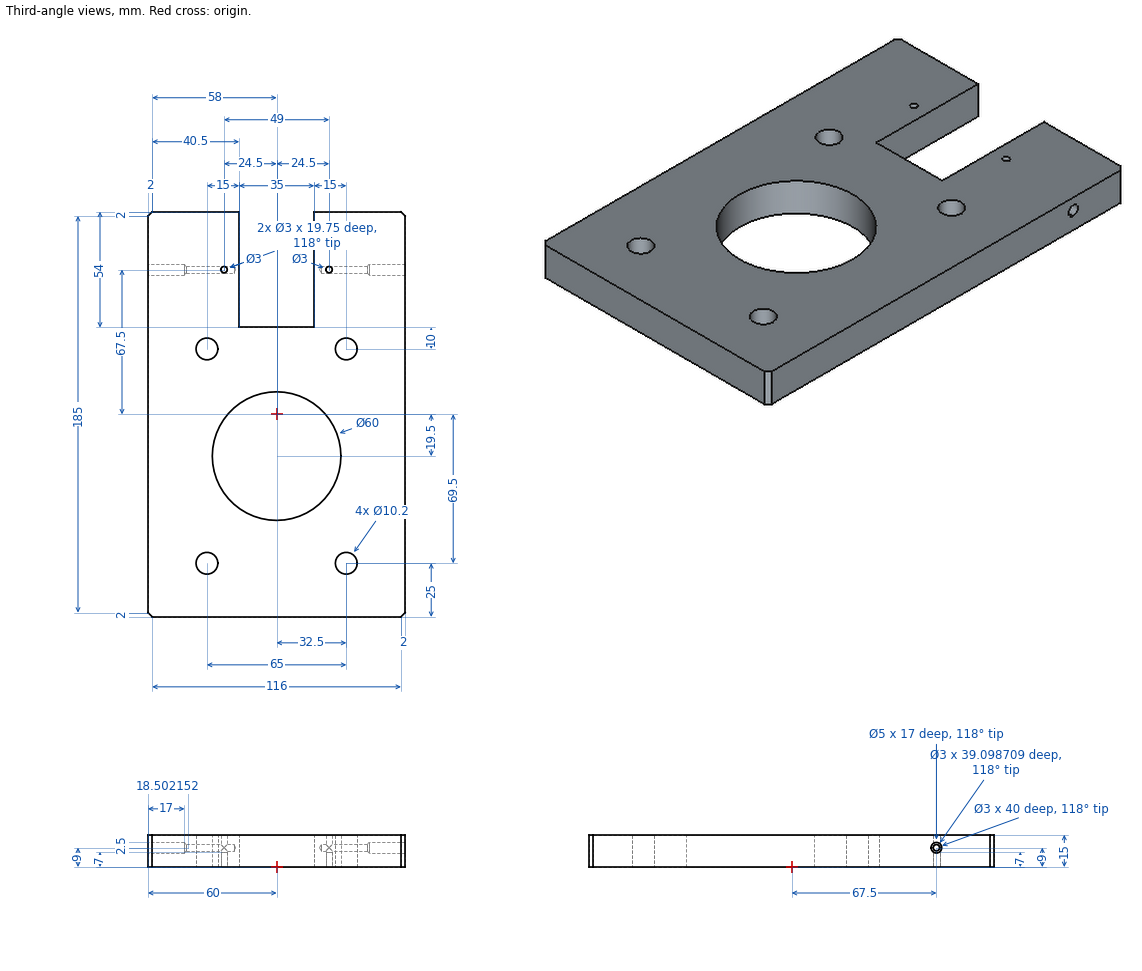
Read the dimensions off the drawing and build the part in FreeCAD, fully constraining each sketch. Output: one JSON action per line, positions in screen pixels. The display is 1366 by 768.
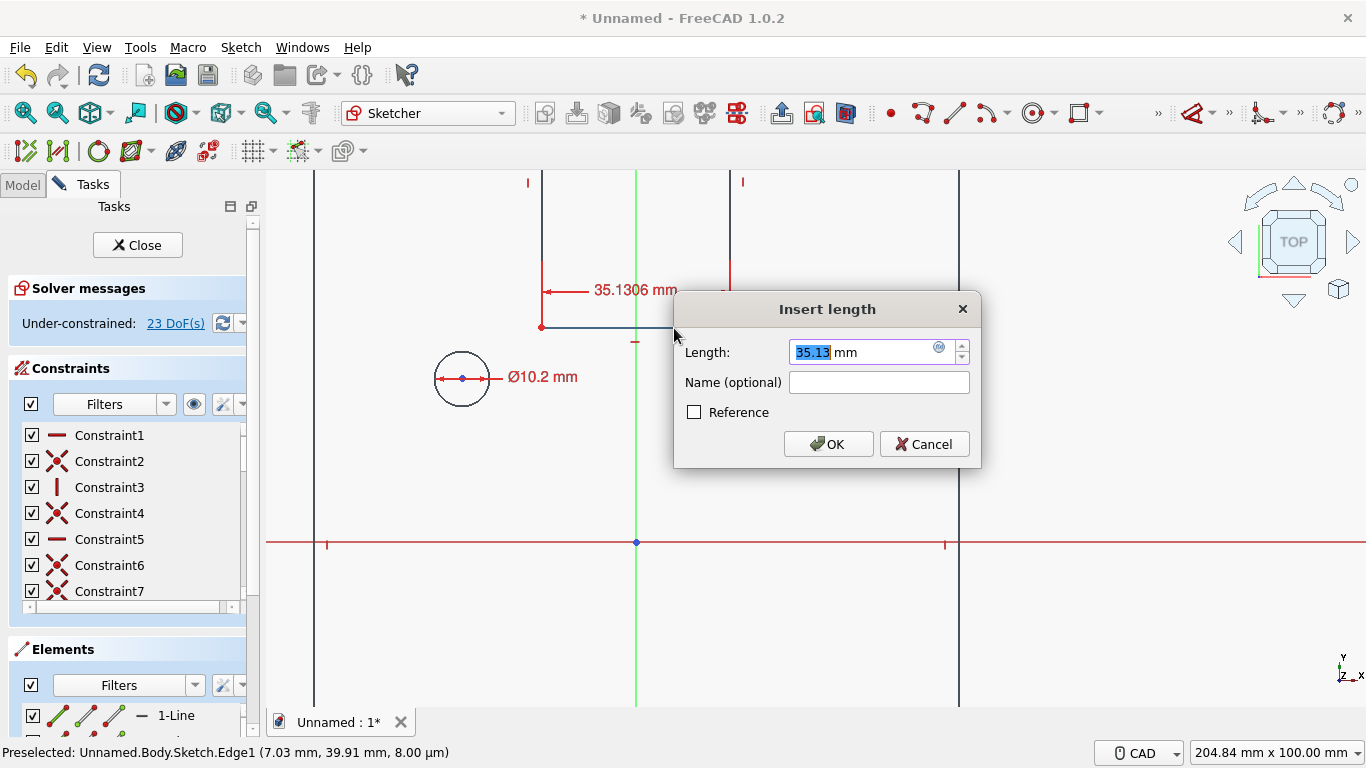
{"action": "type", "text": "35"}
{"action": "key", "text": "Return"}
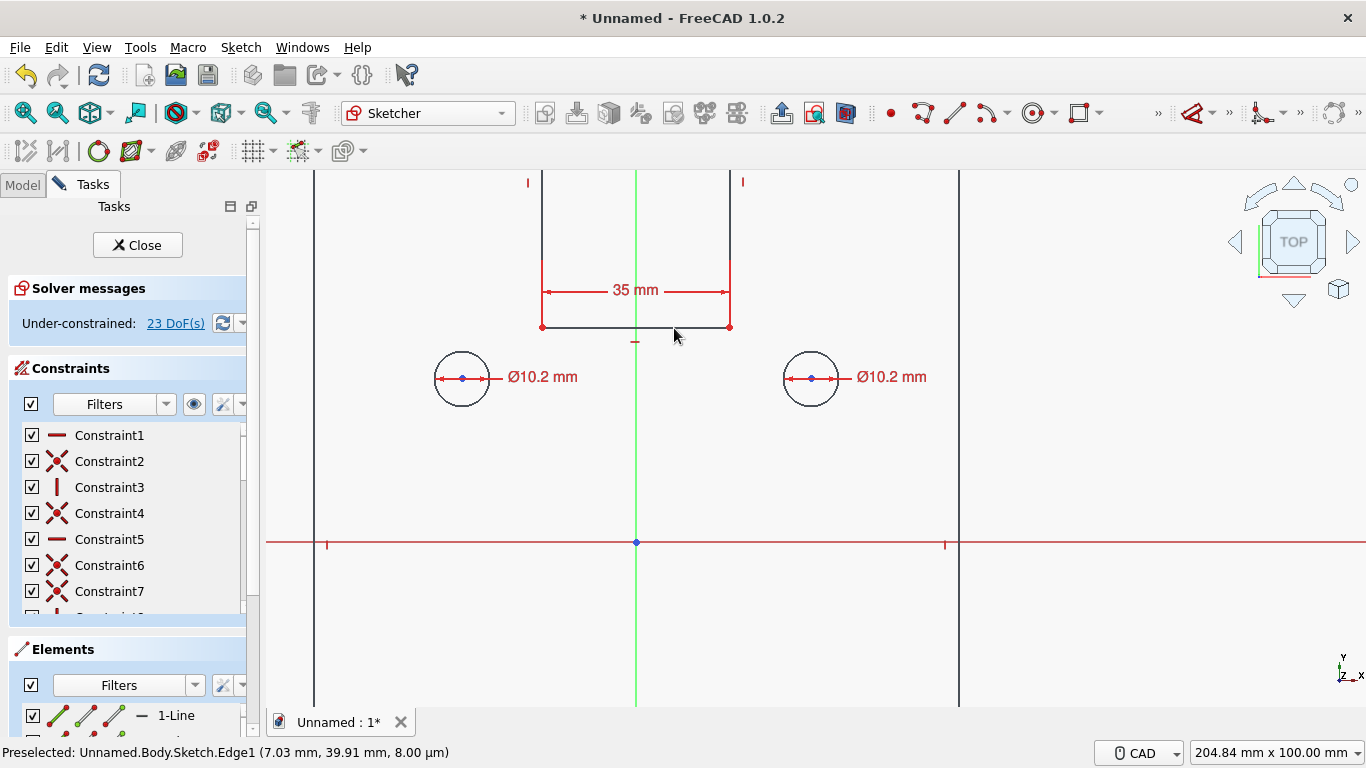
{"action": "left_click", "coordinate": [542, 241]}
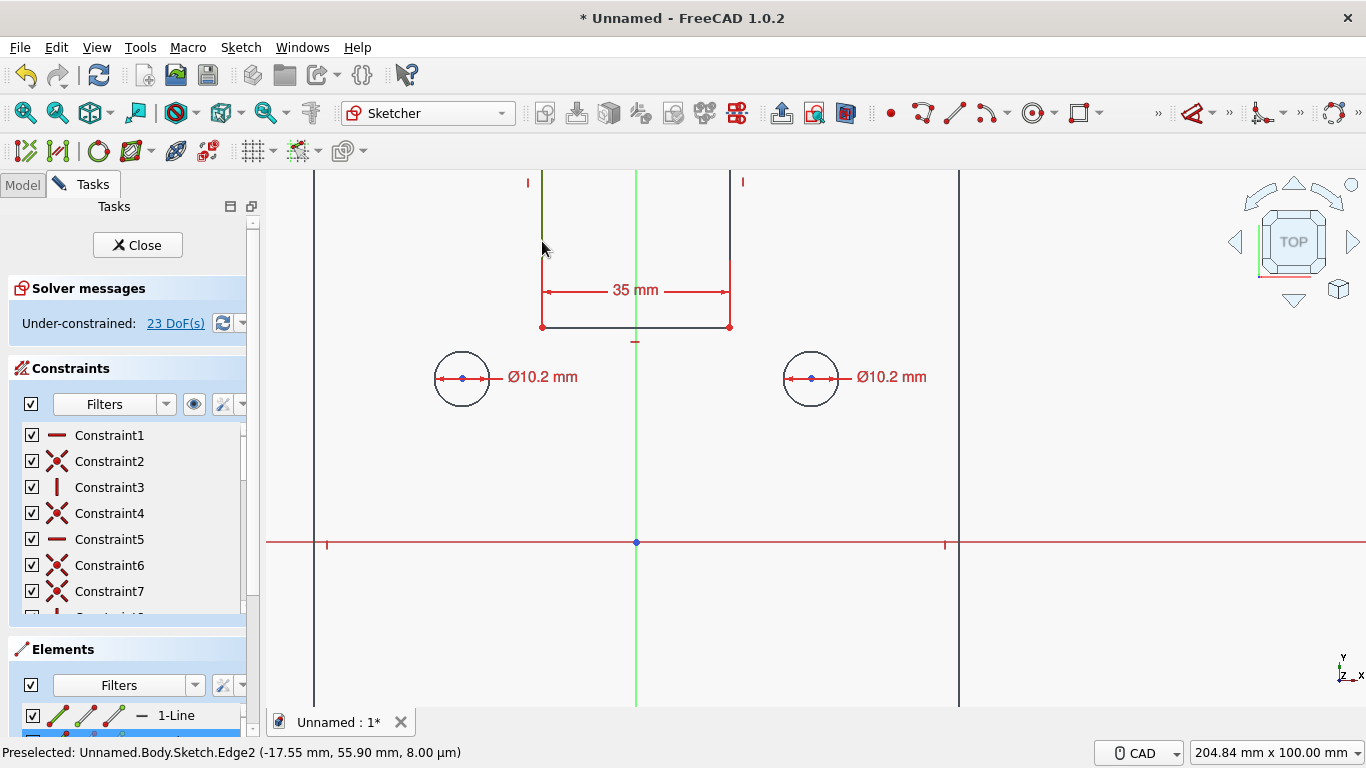
{"action": "key", "text": "i"}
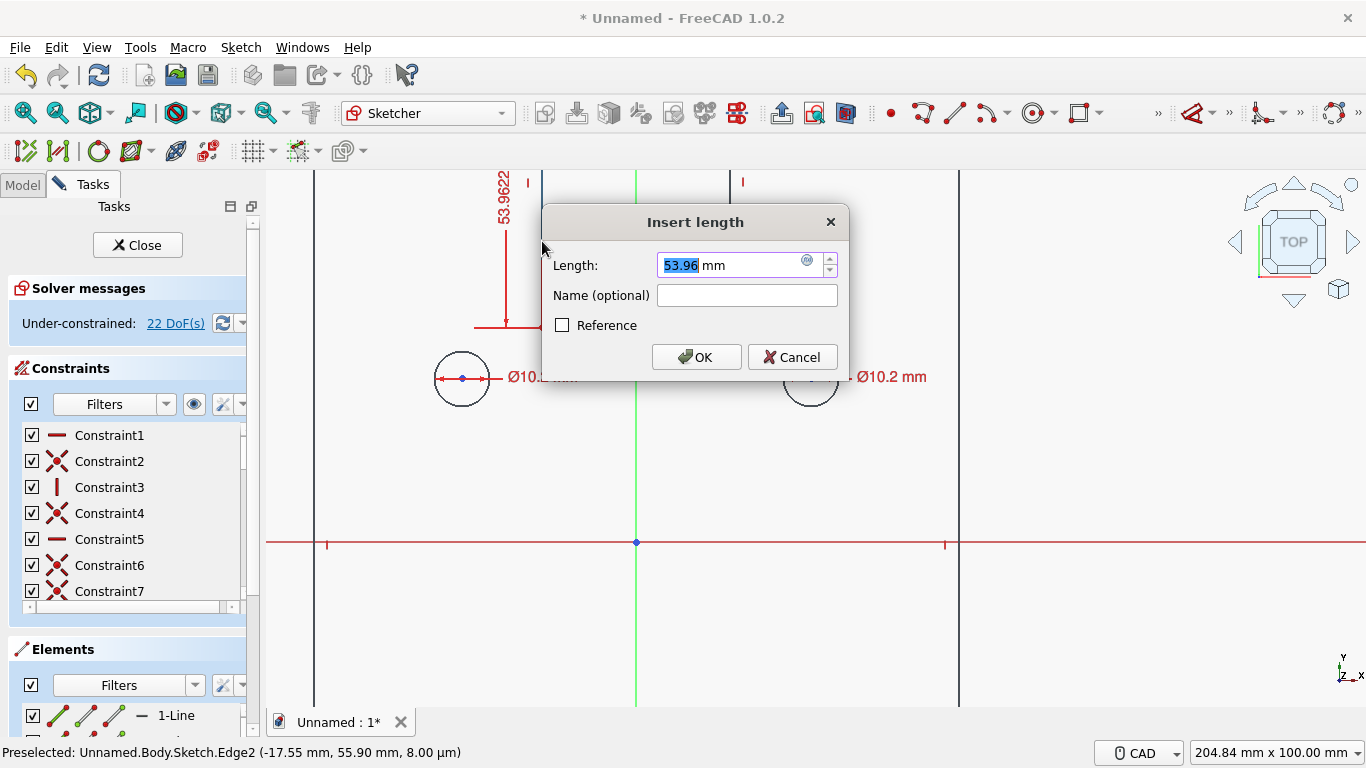
{"action": "type", "text": "54"}
{"action": "key", "text": "Return"}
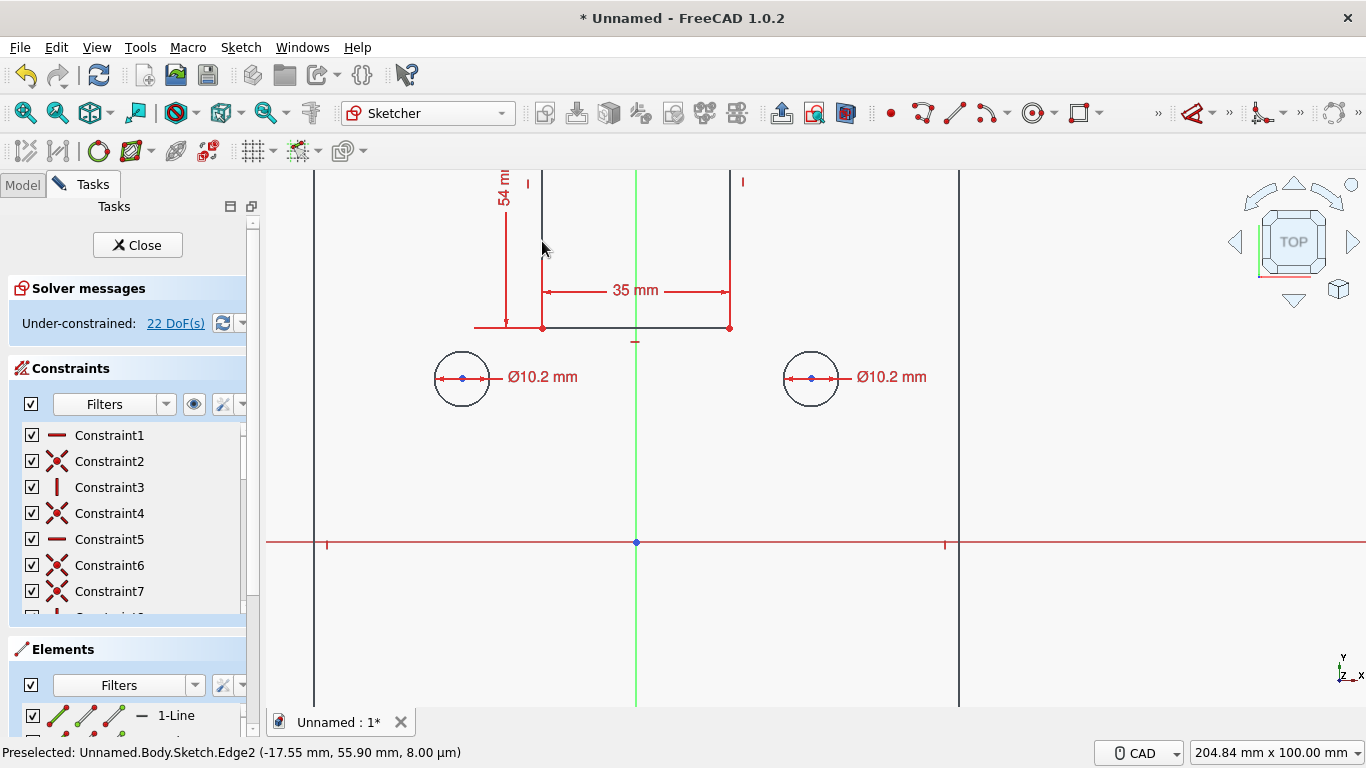
{"action": "left_click", "coordinate": [730, 240]}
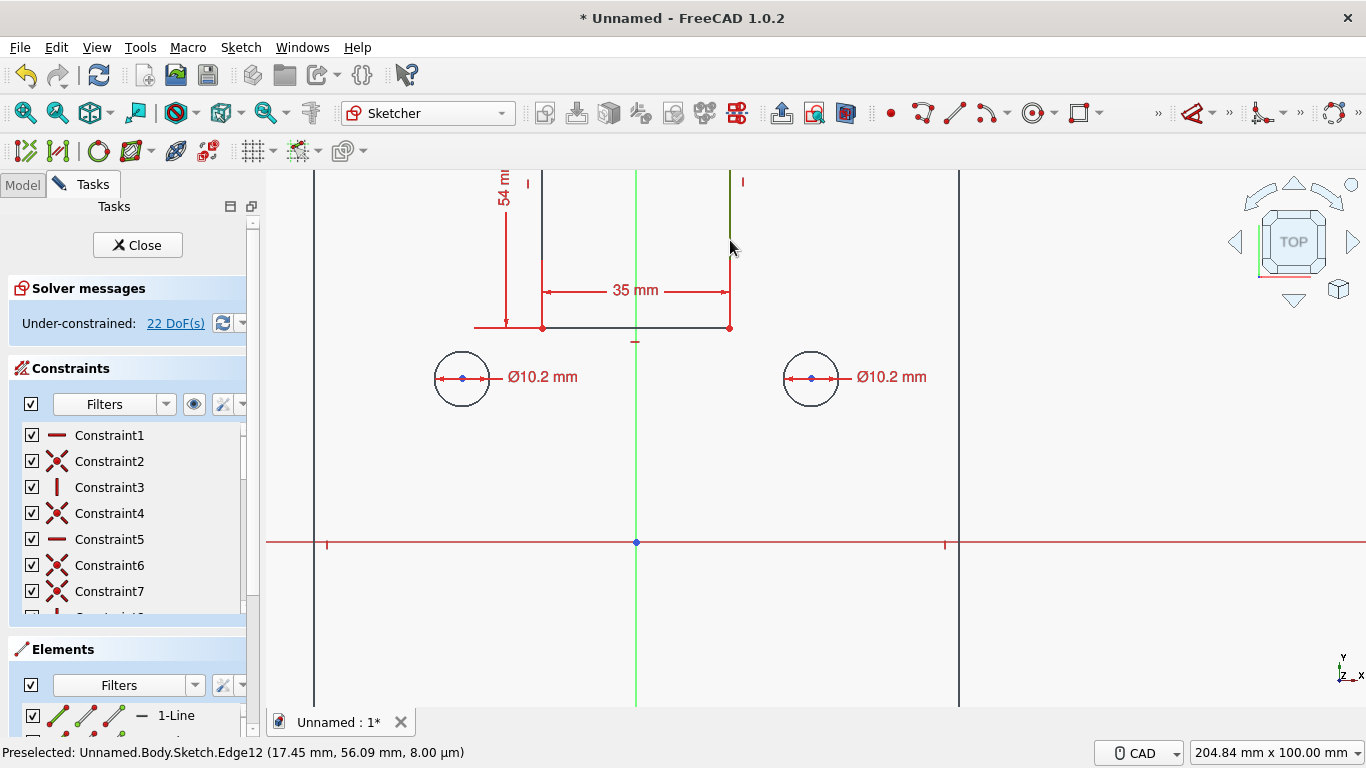
{"action": "key", "text": "i"}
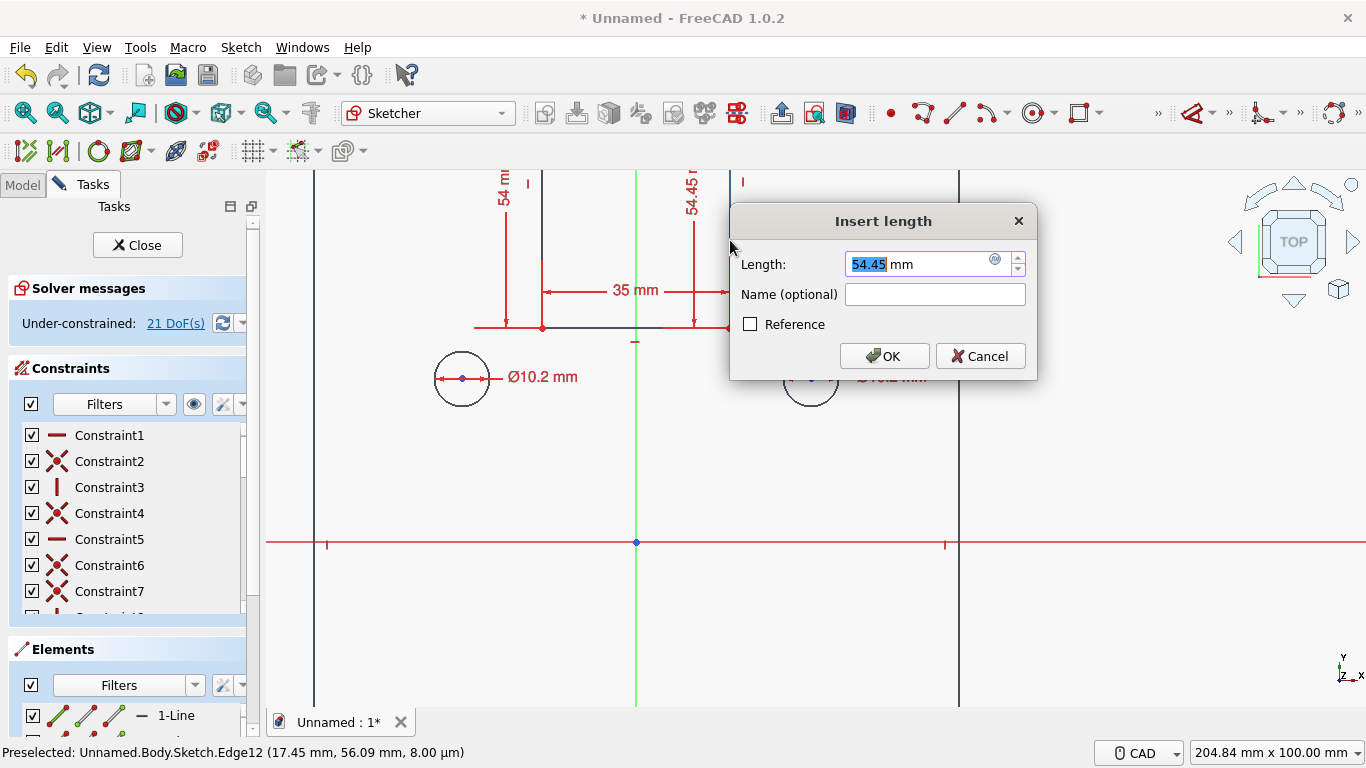
{"action": "type", "text": "54"}
{"action": "key", "text": "Return"}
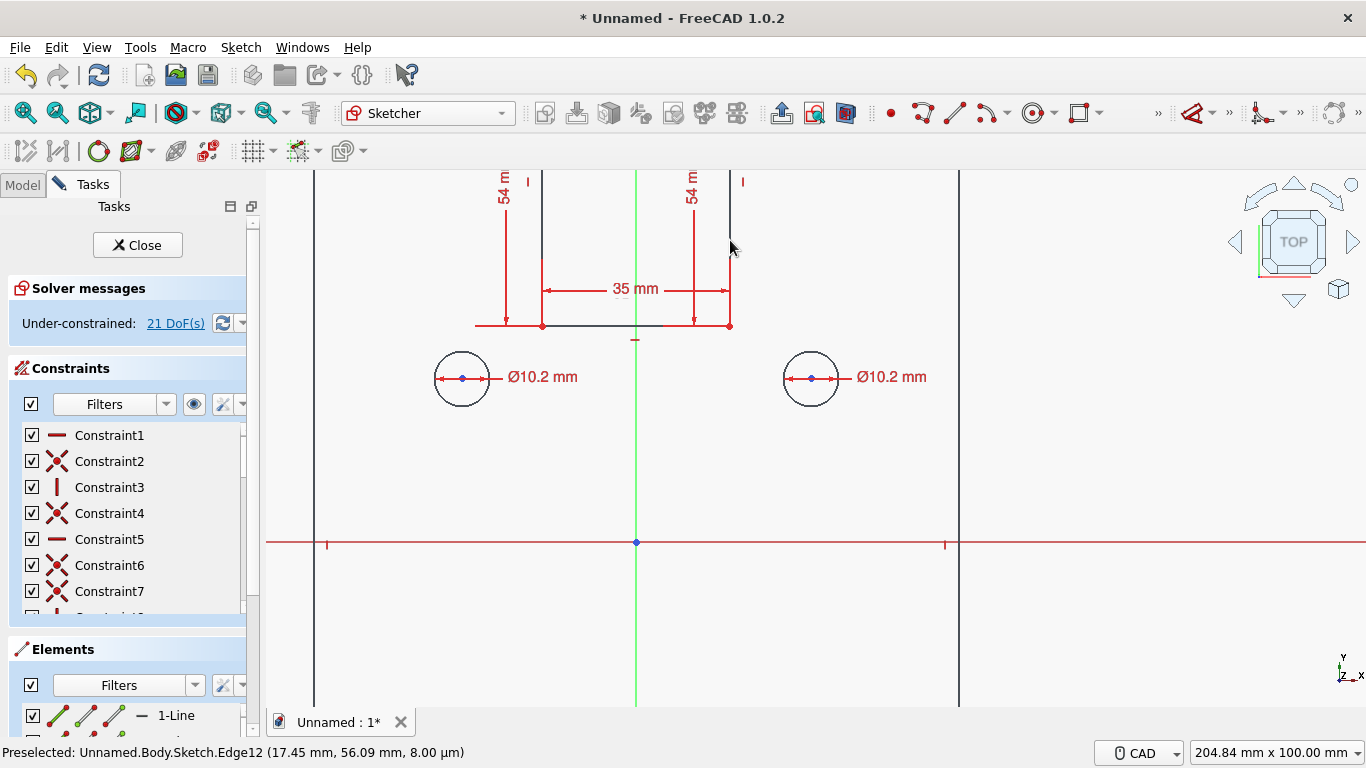
{"action": "scroll", "coordinate": [812, 378], "scroll_direction": "down", "scroll_amount": 5}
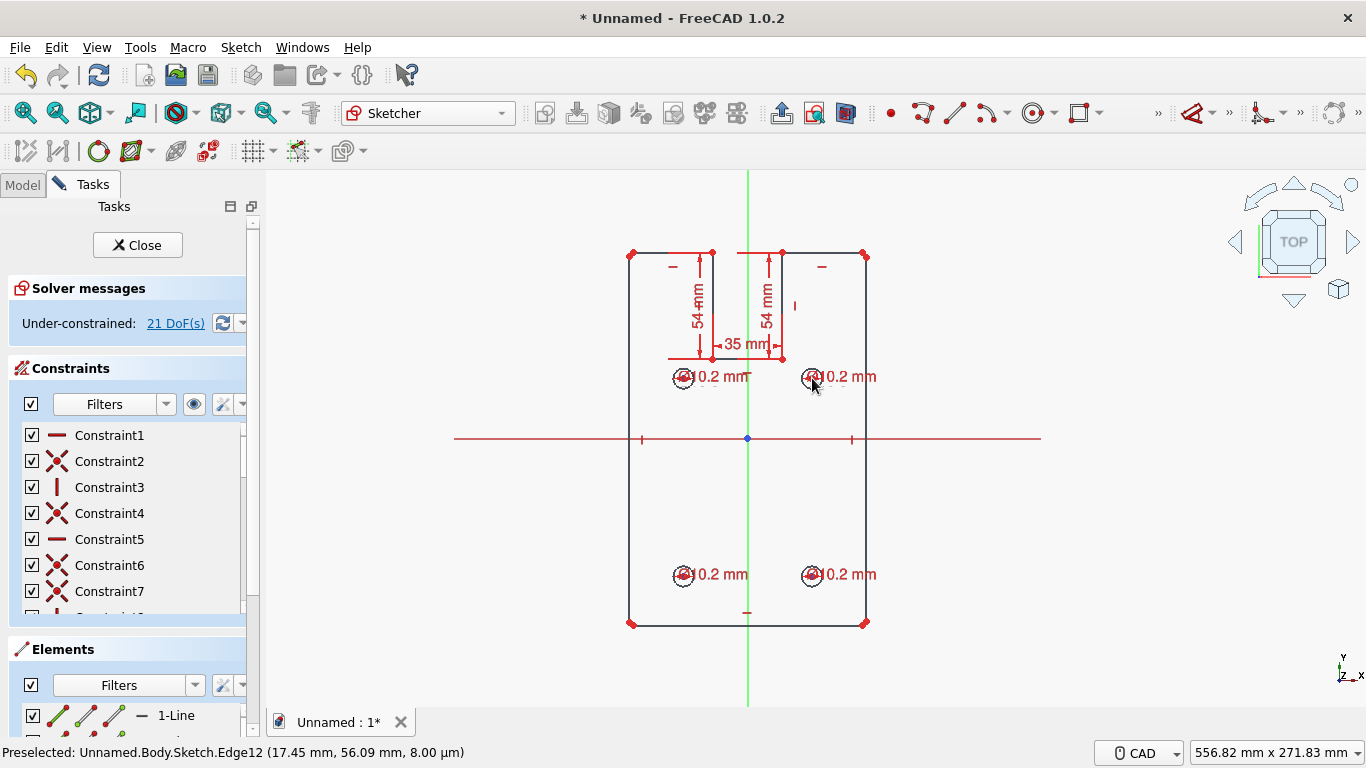
{"action": "scroll", "coordinate": [631, 254], "scroll_direction": "up", "scroll_amount": 12}